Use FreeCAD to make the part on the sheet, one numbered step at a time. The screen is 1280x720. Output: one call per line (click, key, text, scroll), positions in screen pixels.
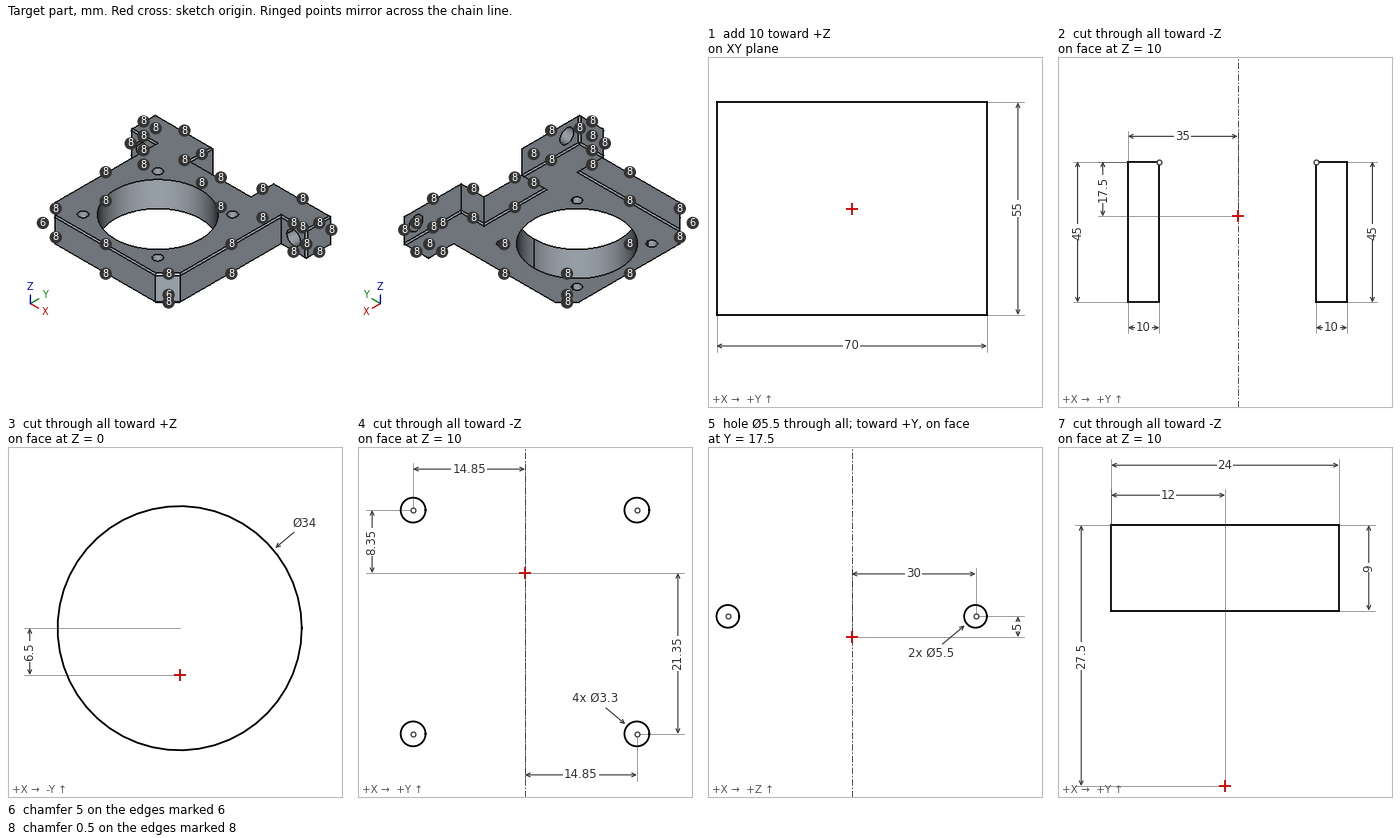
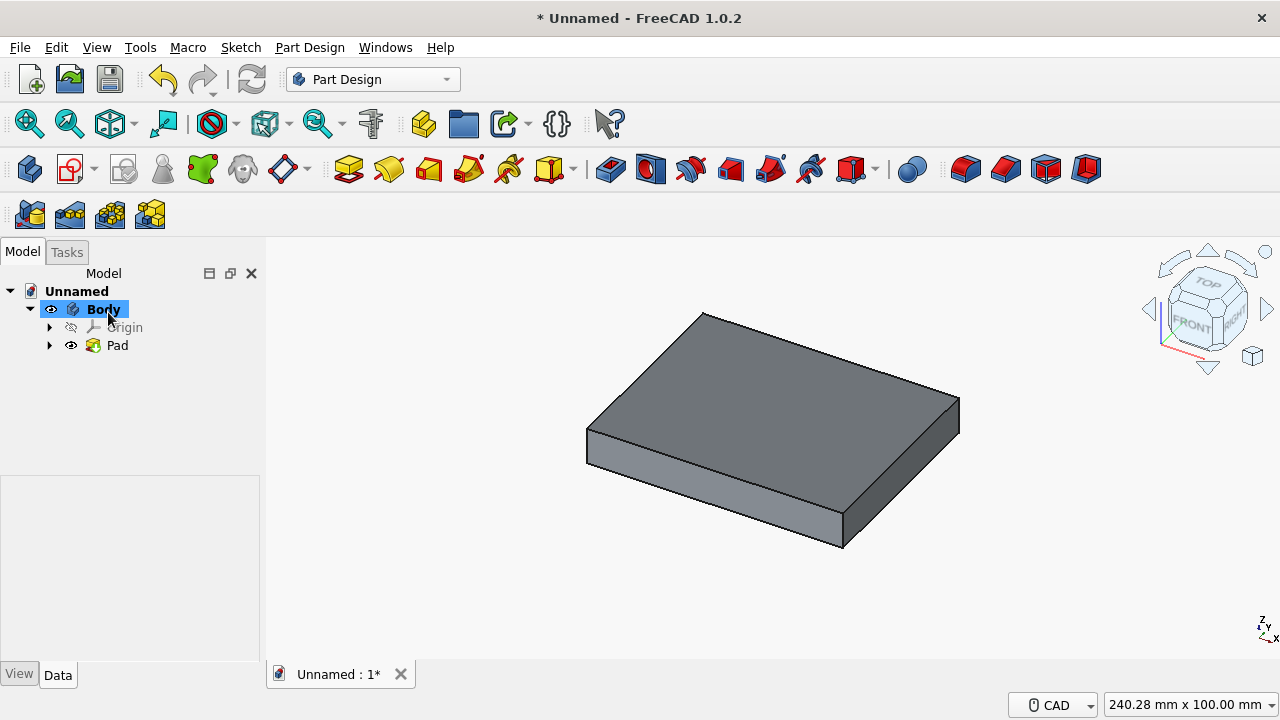
click(773, 412)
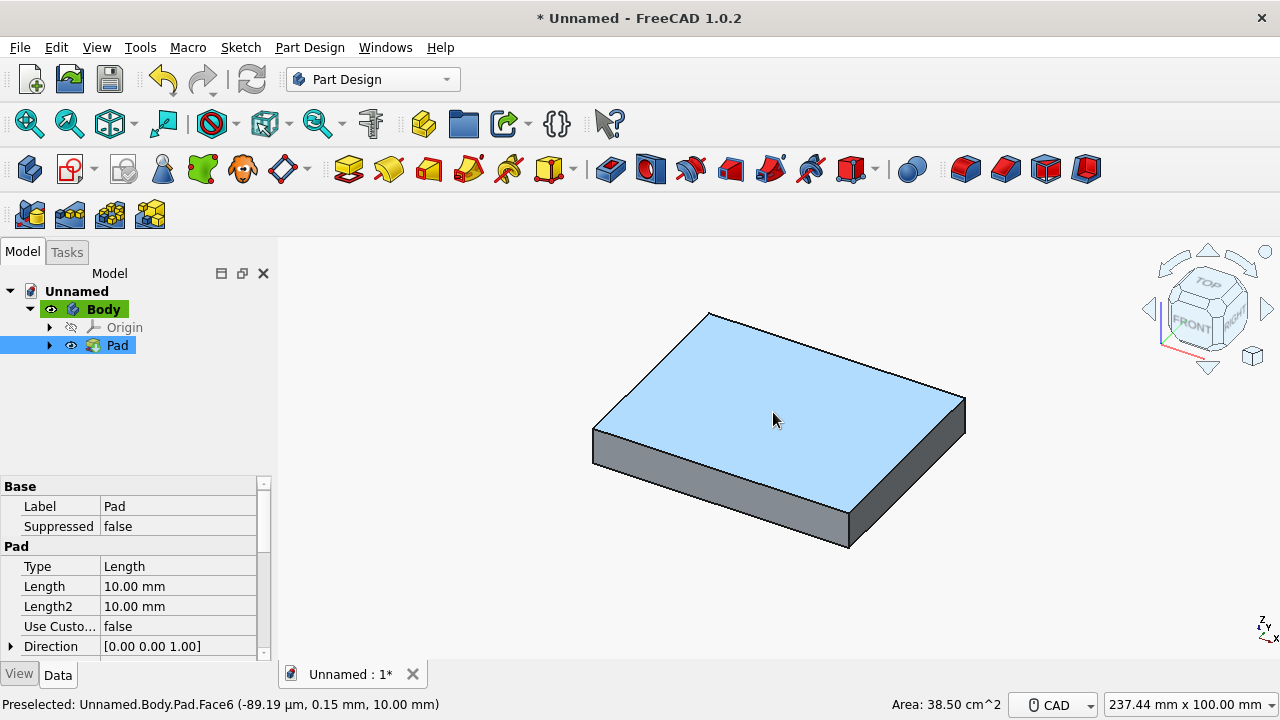
click(70, 170)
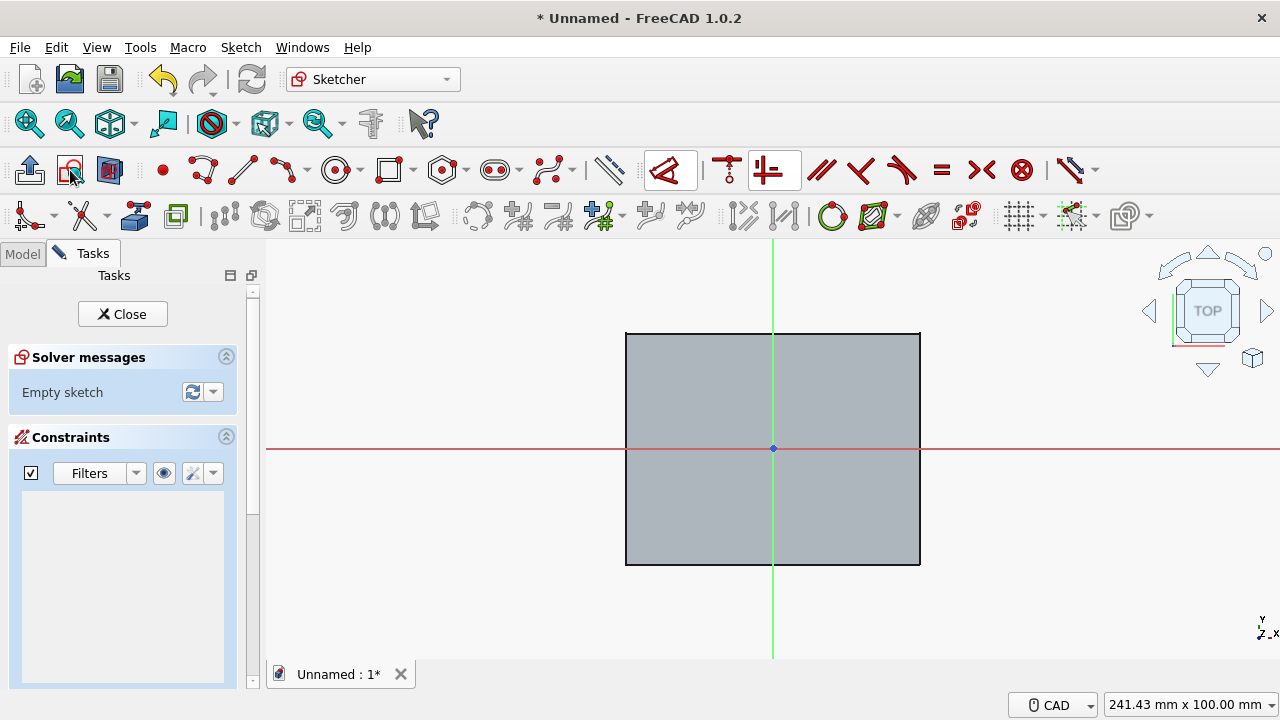
scroll(912, 513, up, 2)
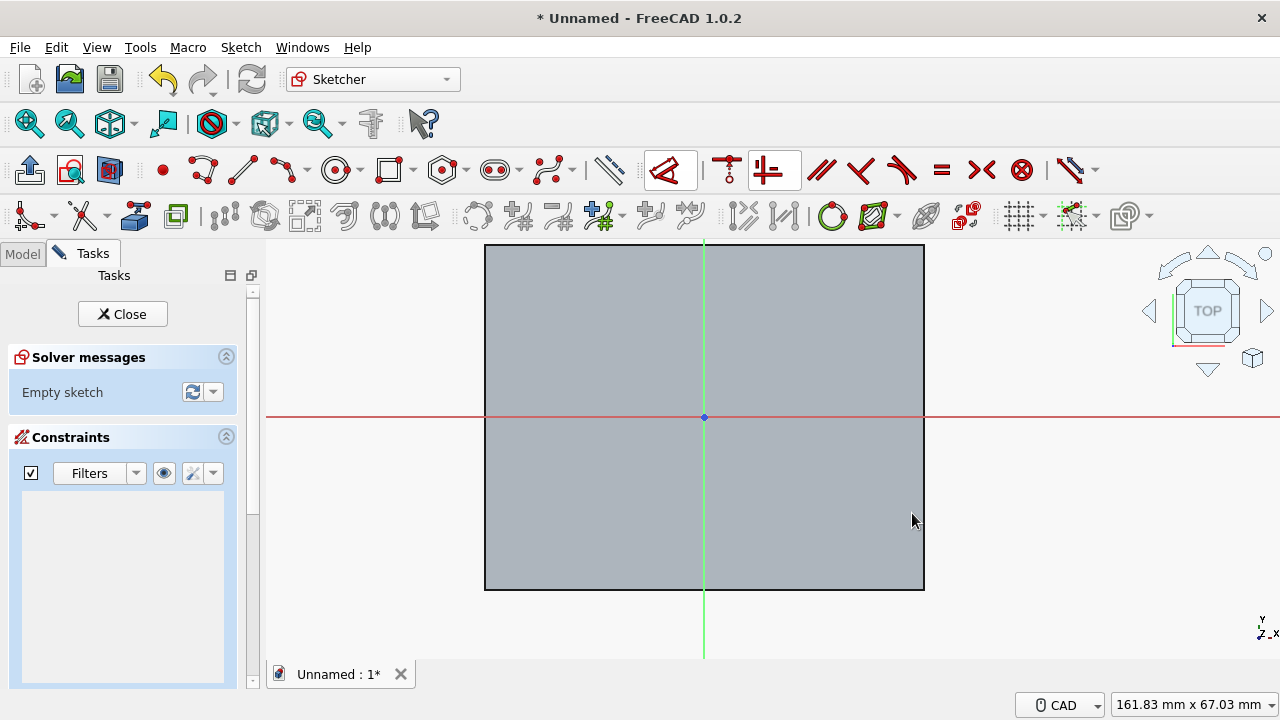
click(390, 170)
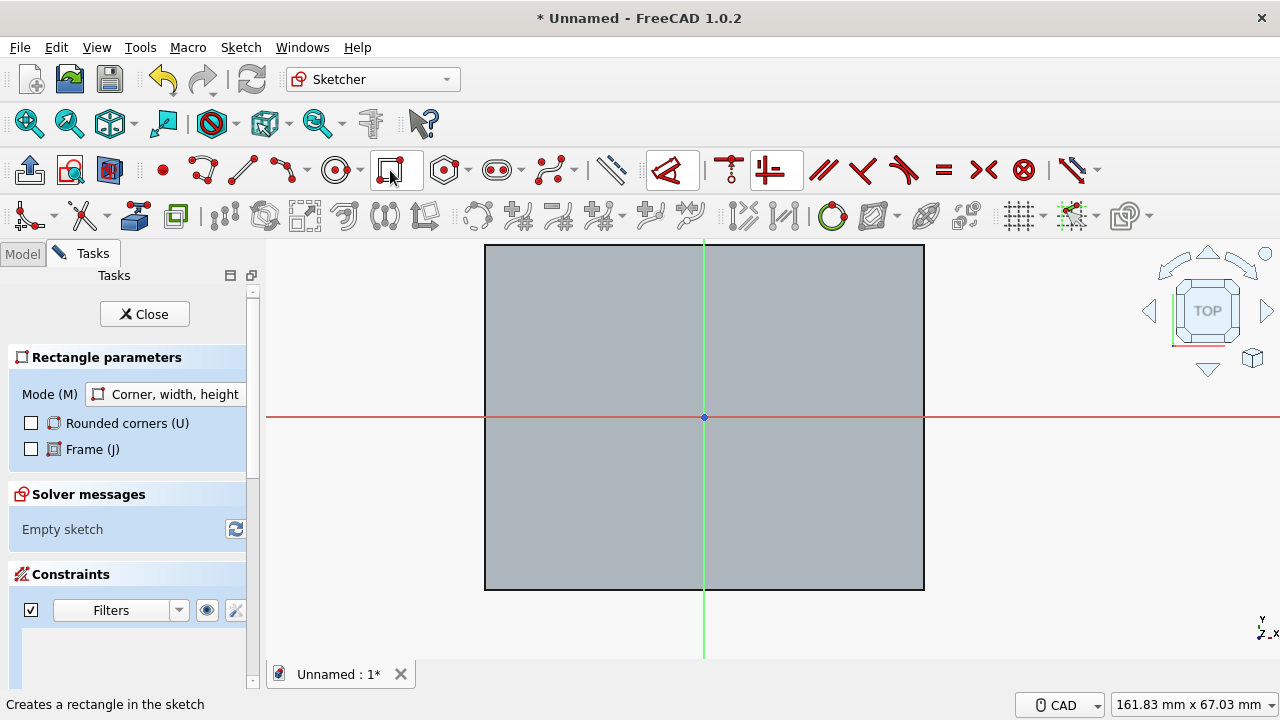
click(485, 308)
move(548, 590)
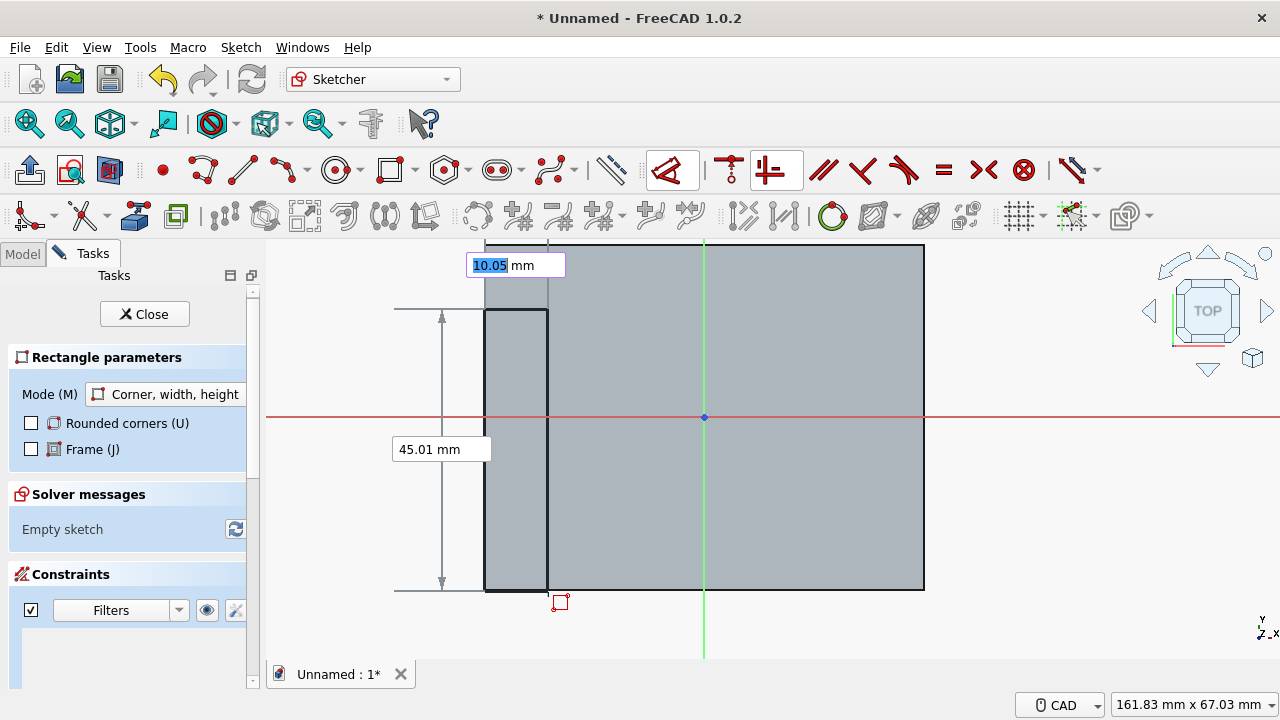
text(10)
key(Tab)
text(45)
key(Return)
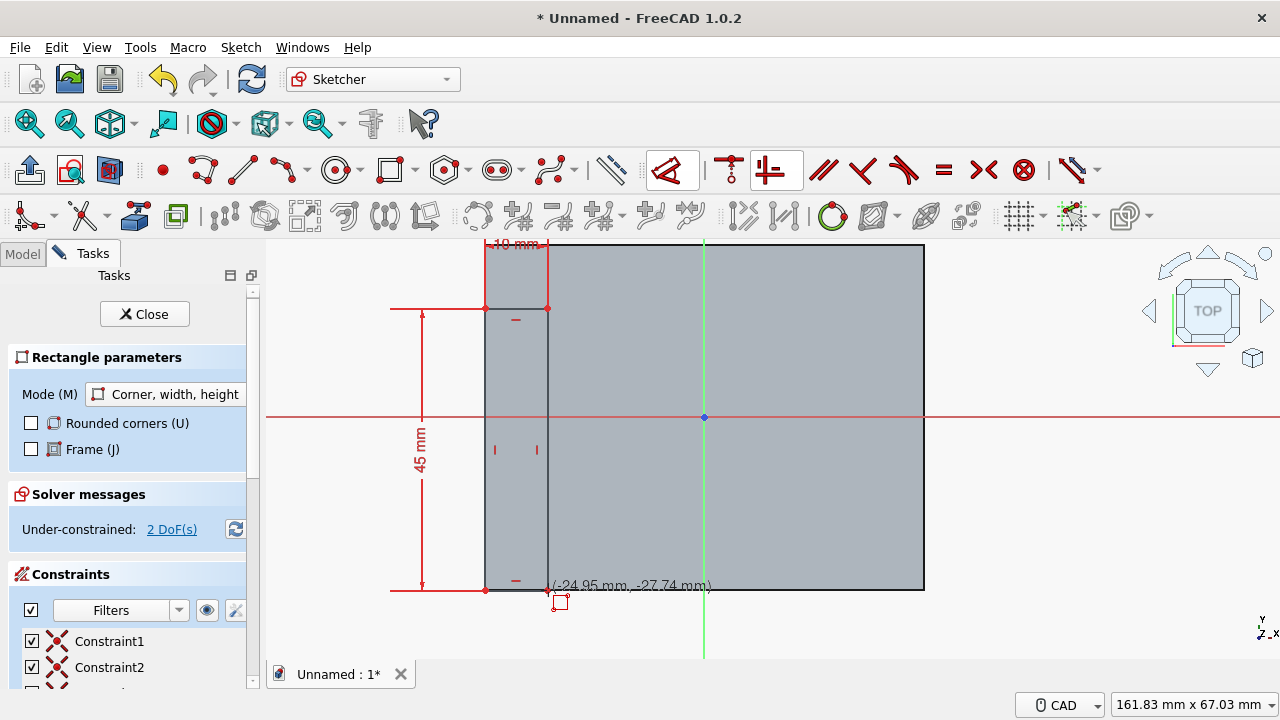
click(861, 308)
move(924, 590)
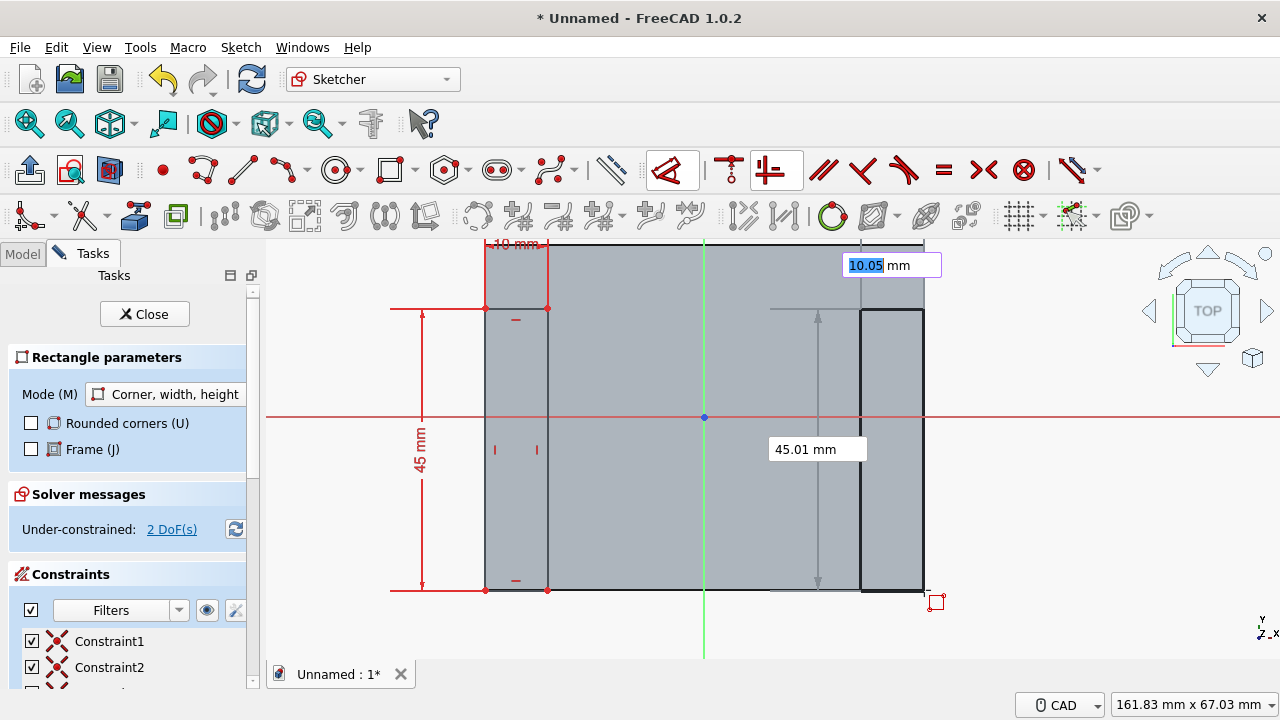
text(10)
key(Tab)
text(45)
key(Return)
key(Escape)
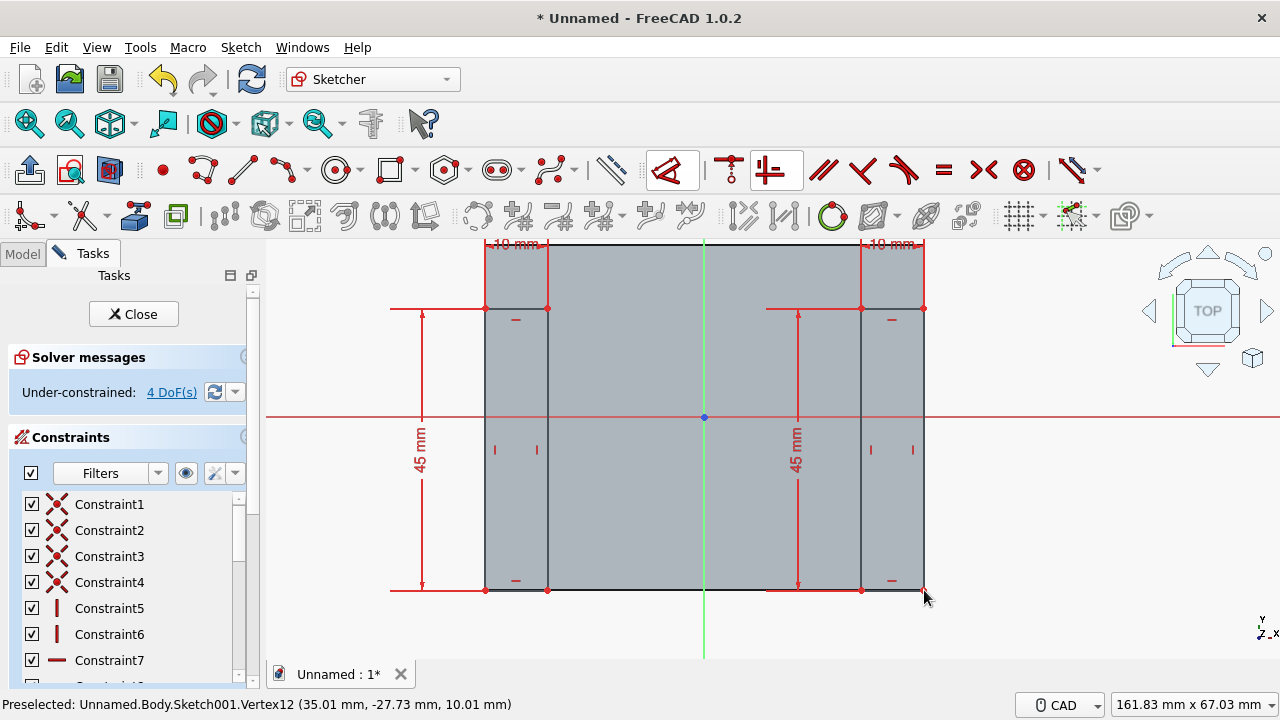
click(548, 309)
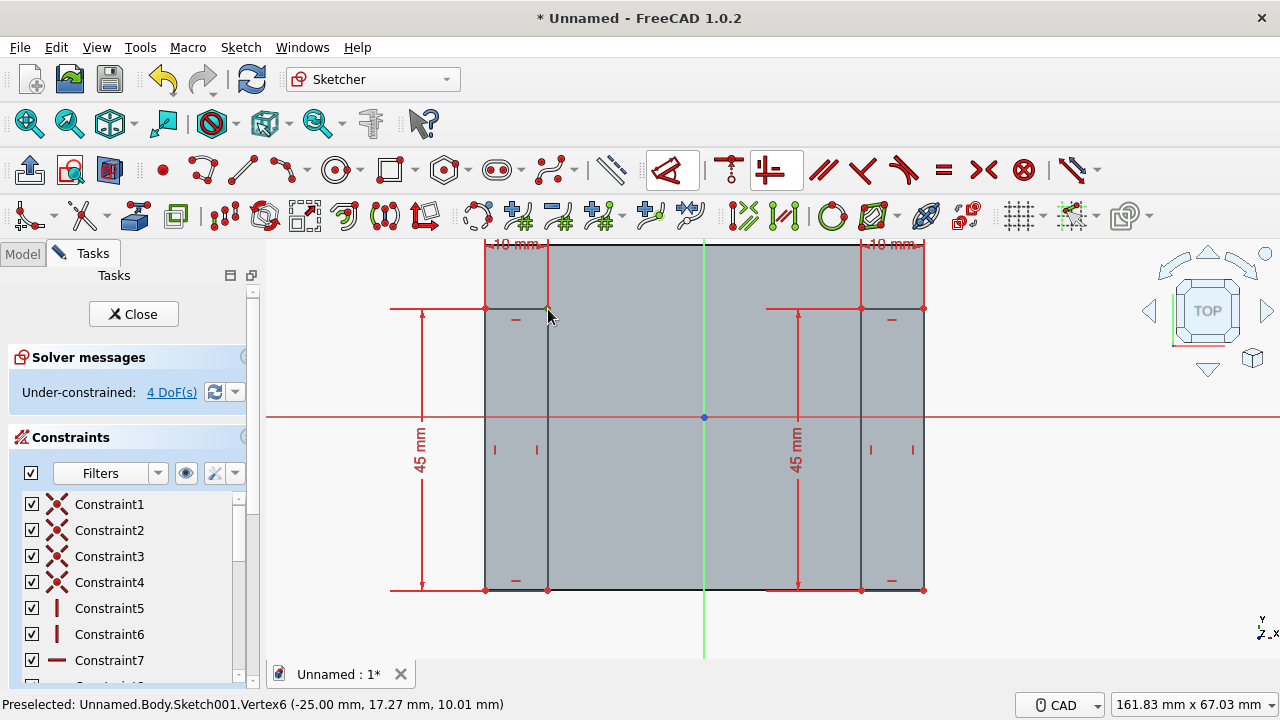
click(861, 309)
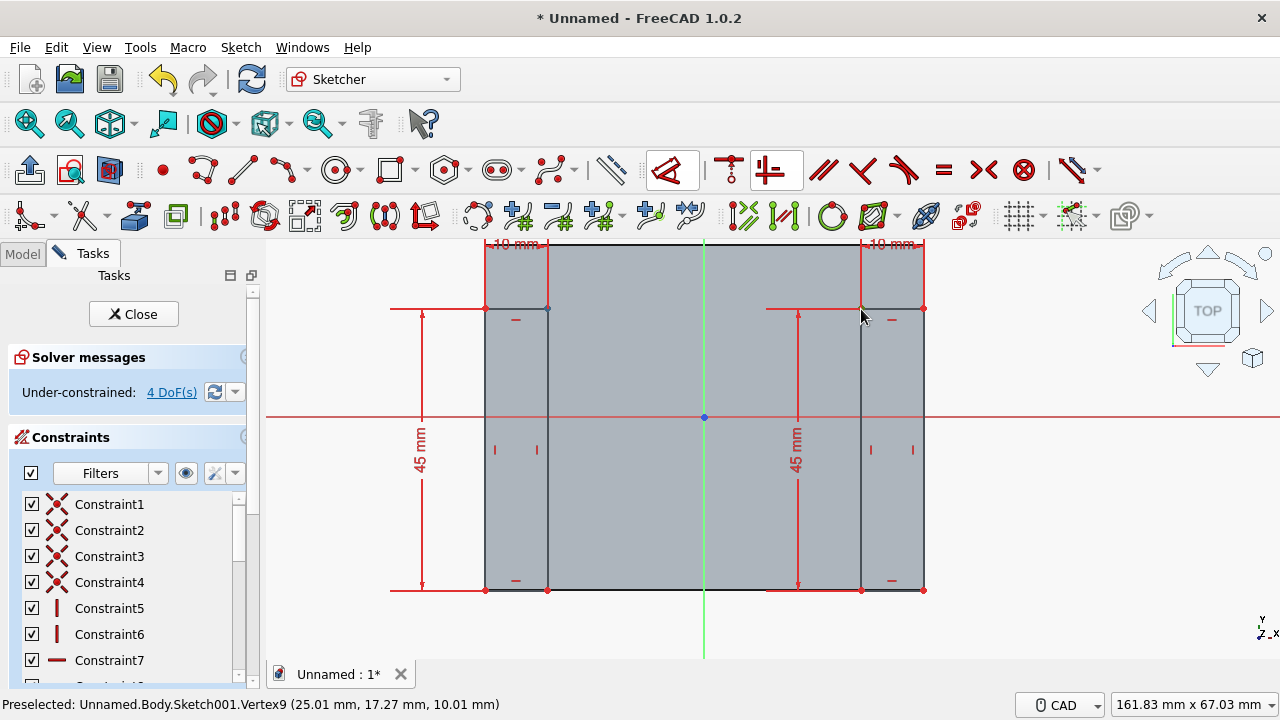
click(704, 605)